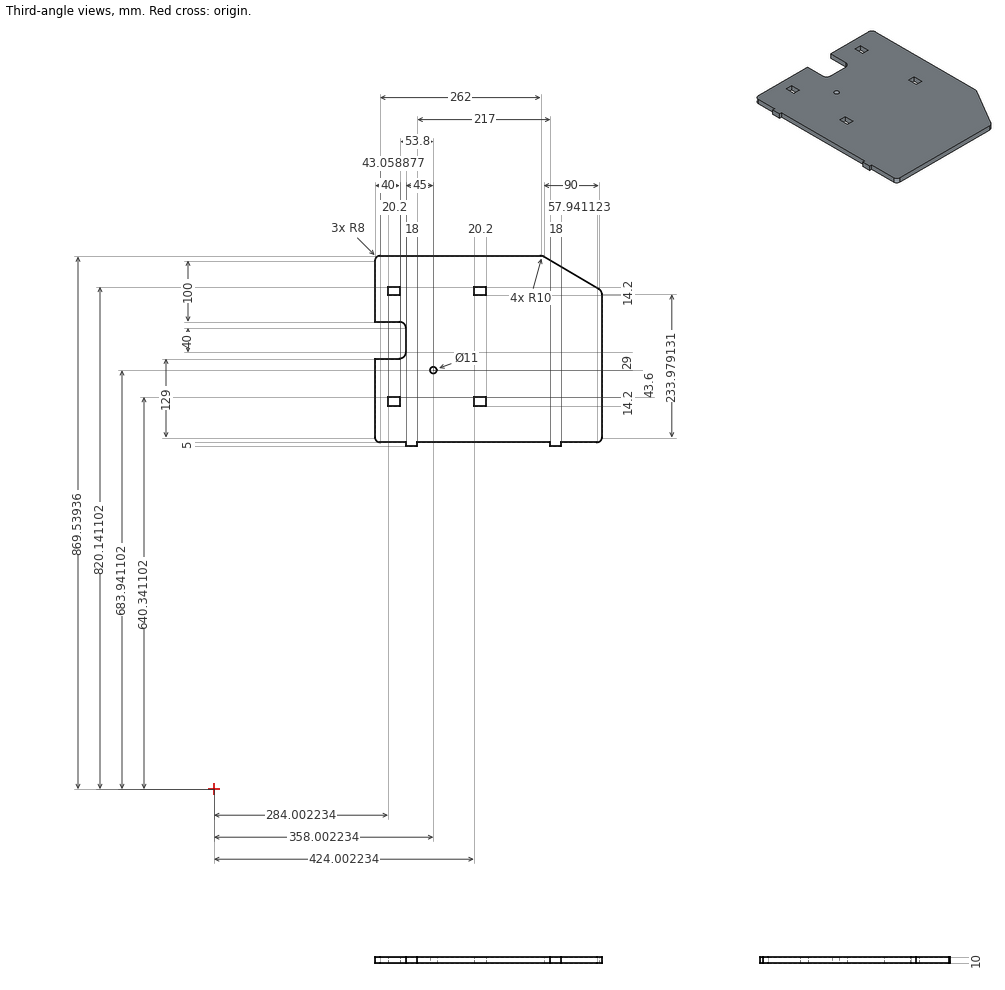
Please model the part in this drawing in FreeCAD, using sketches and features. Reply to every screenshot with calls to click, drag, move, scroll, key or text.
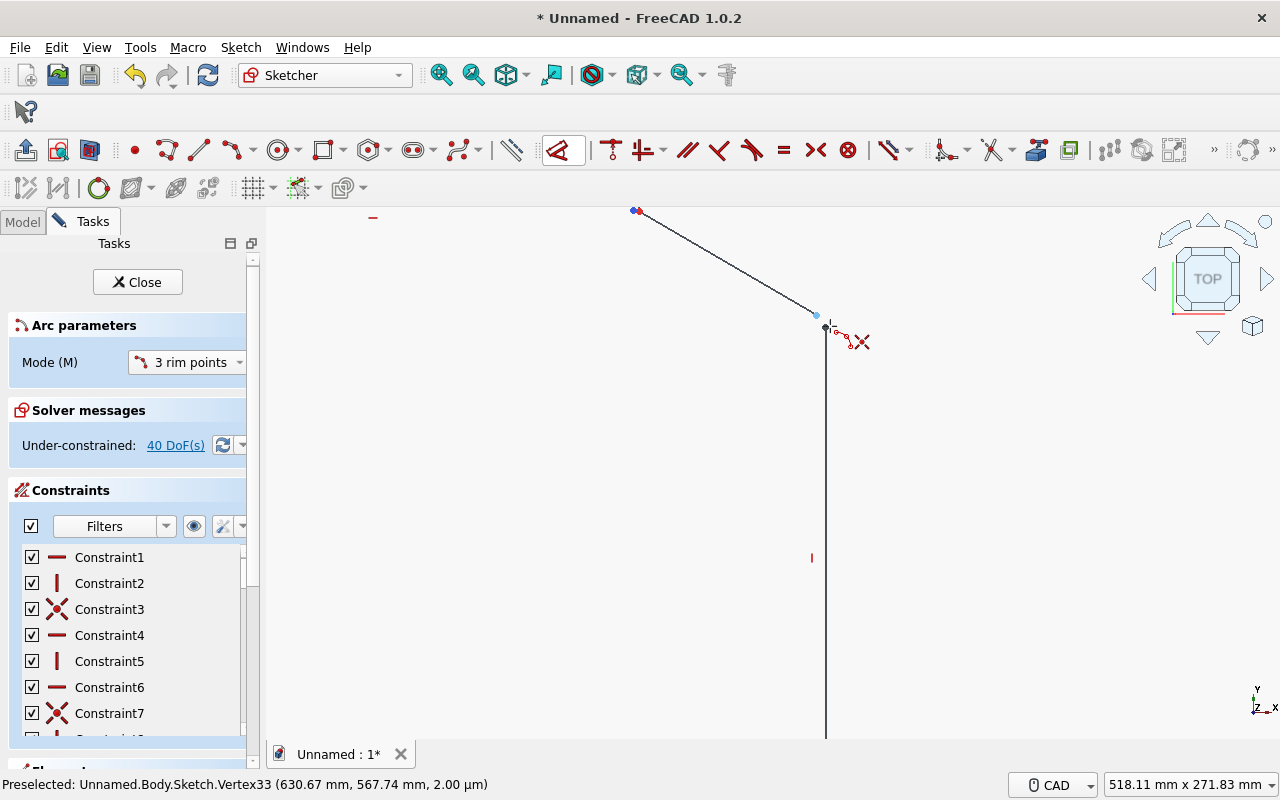
click(826, 328)
click(817, 315)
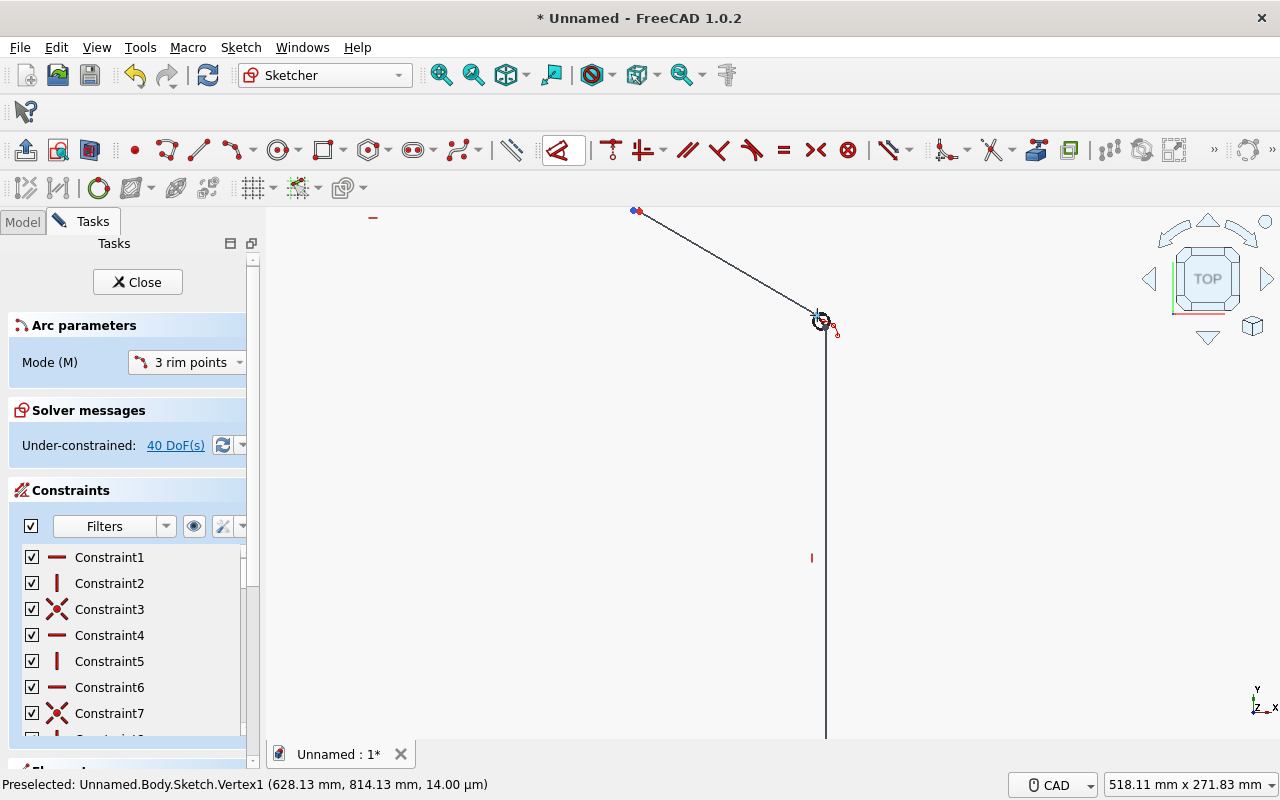
scroll(824, 318, up, 10)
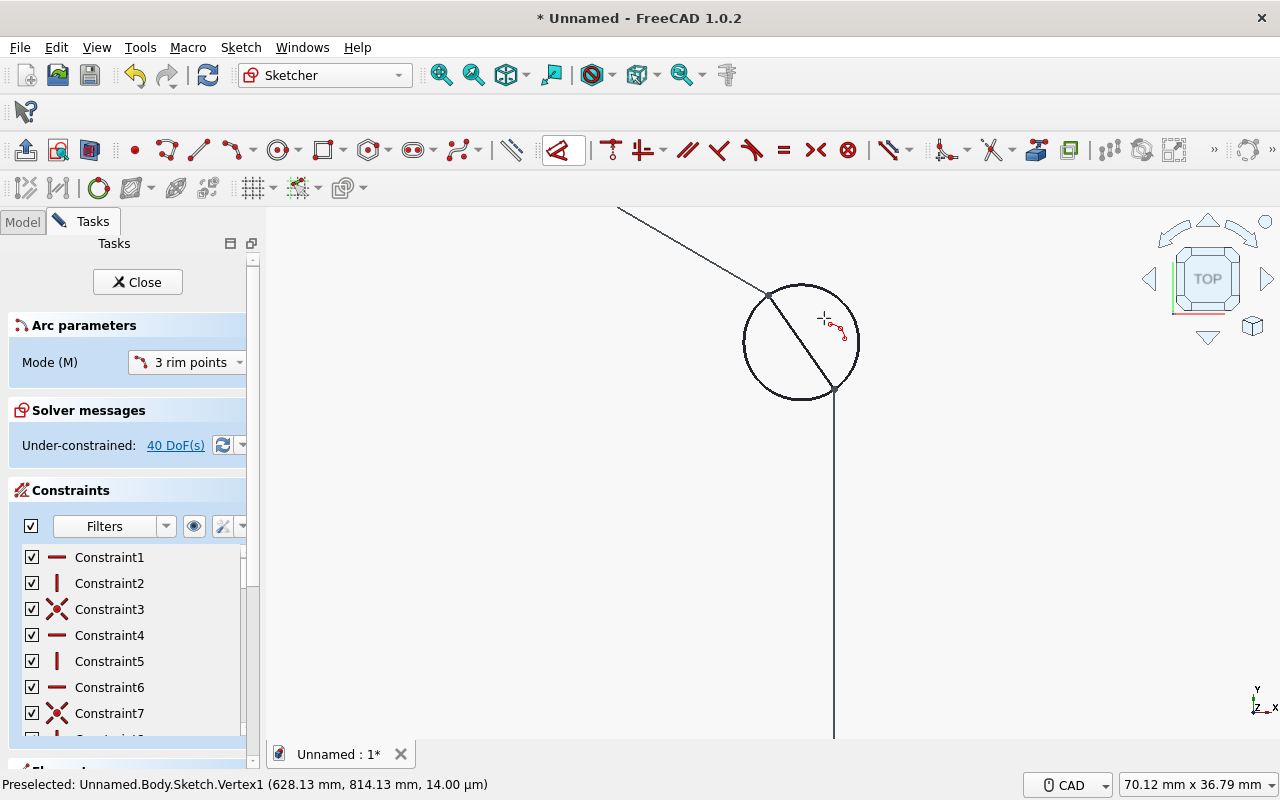
click(820, 313)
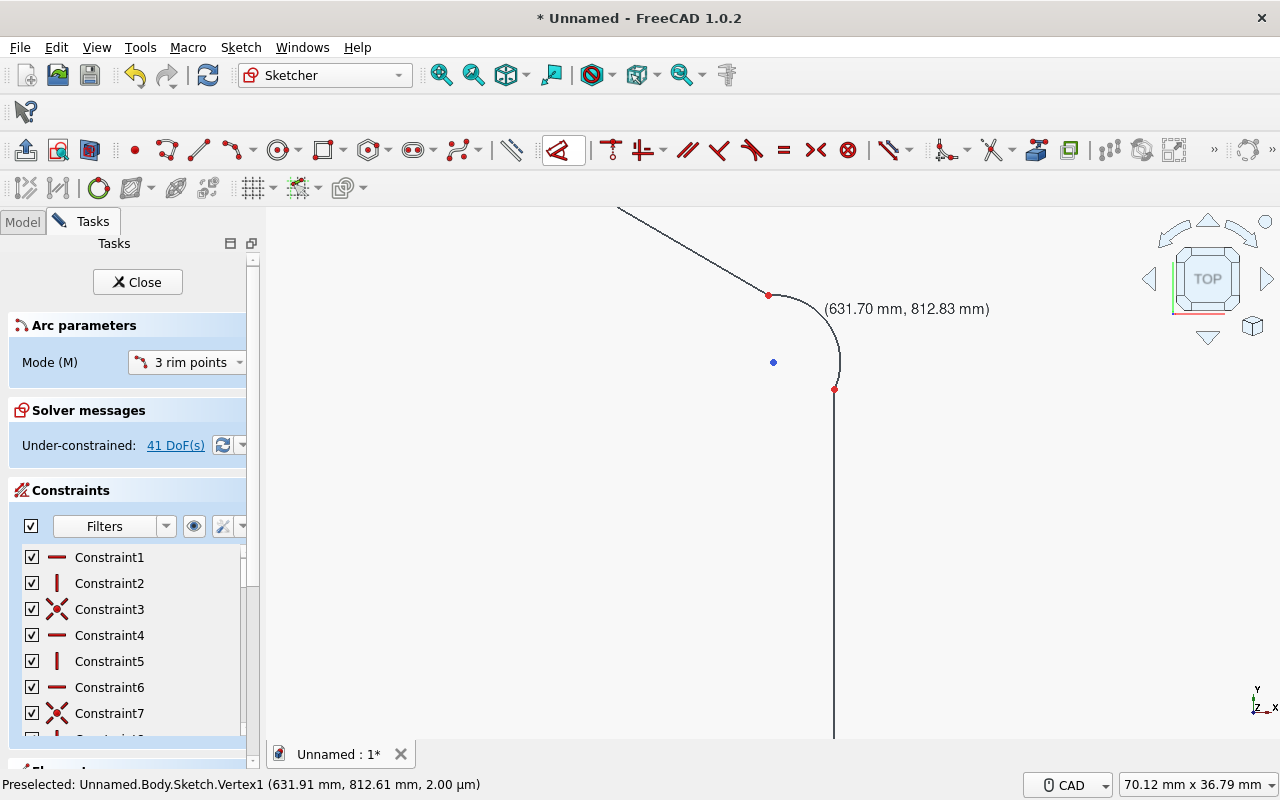
click(324, 150)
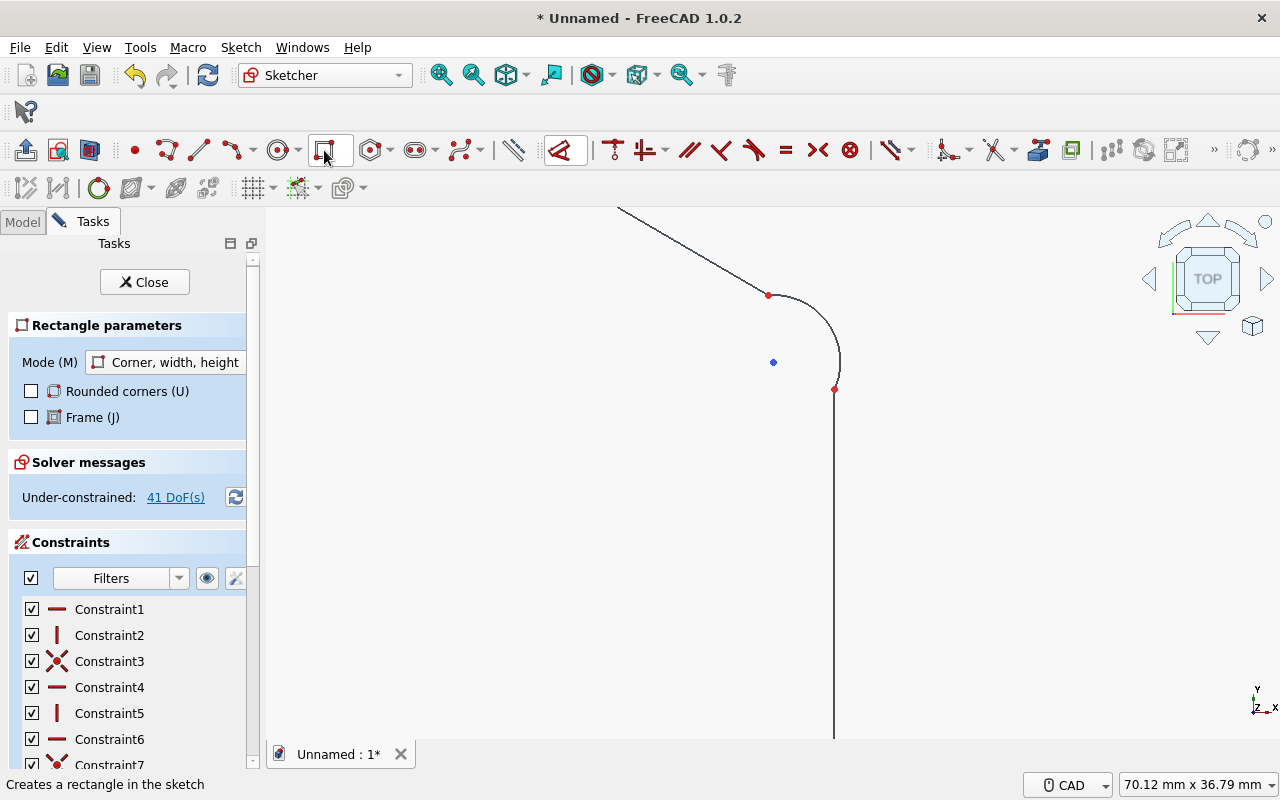
scroll(858, 290, down, 17)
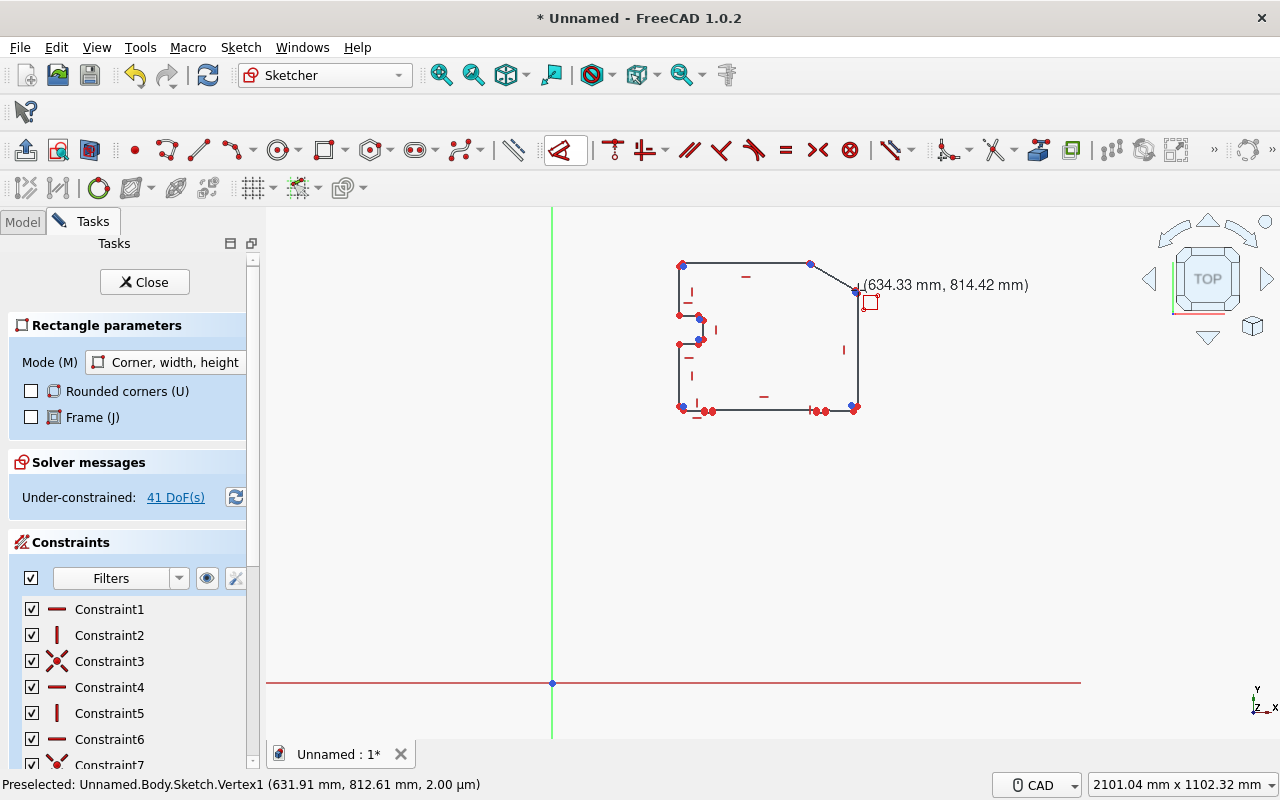
scroll(757, 374, up, 5)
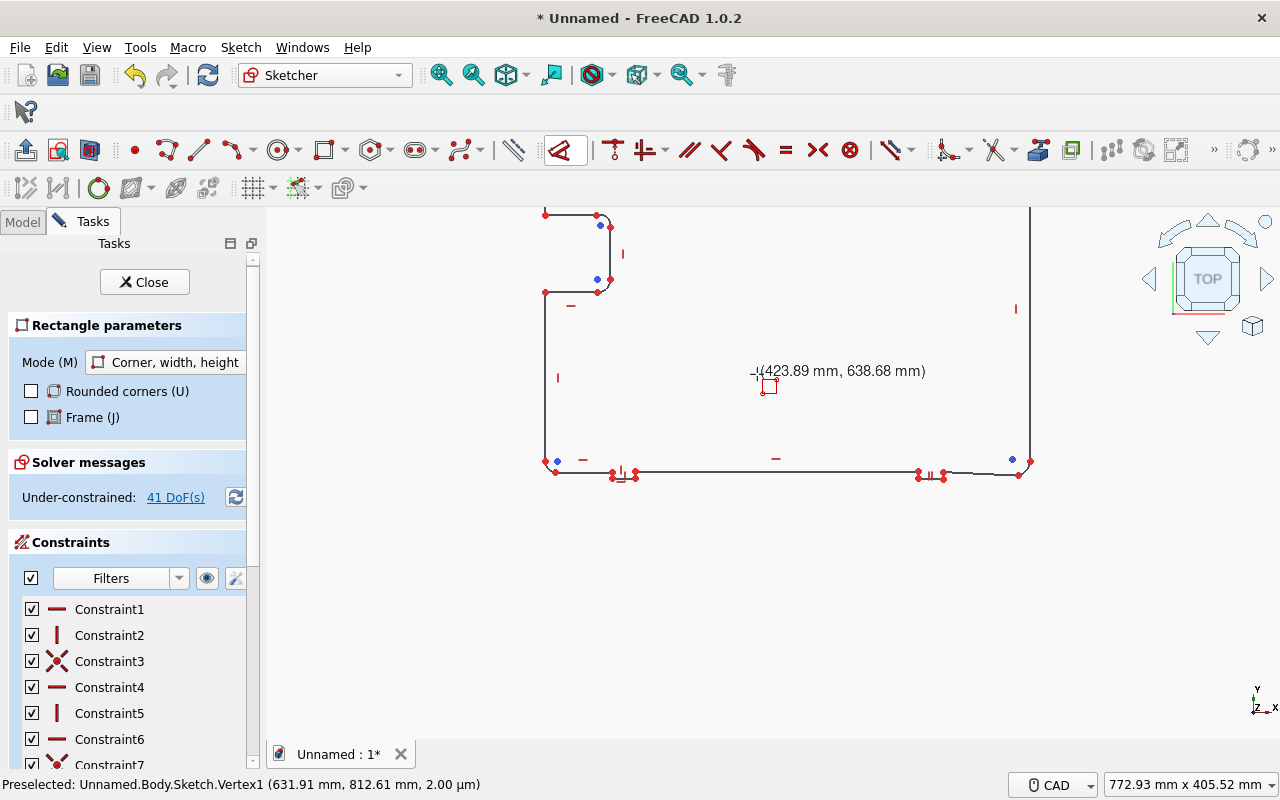
click(756, 374)
move(783, 393)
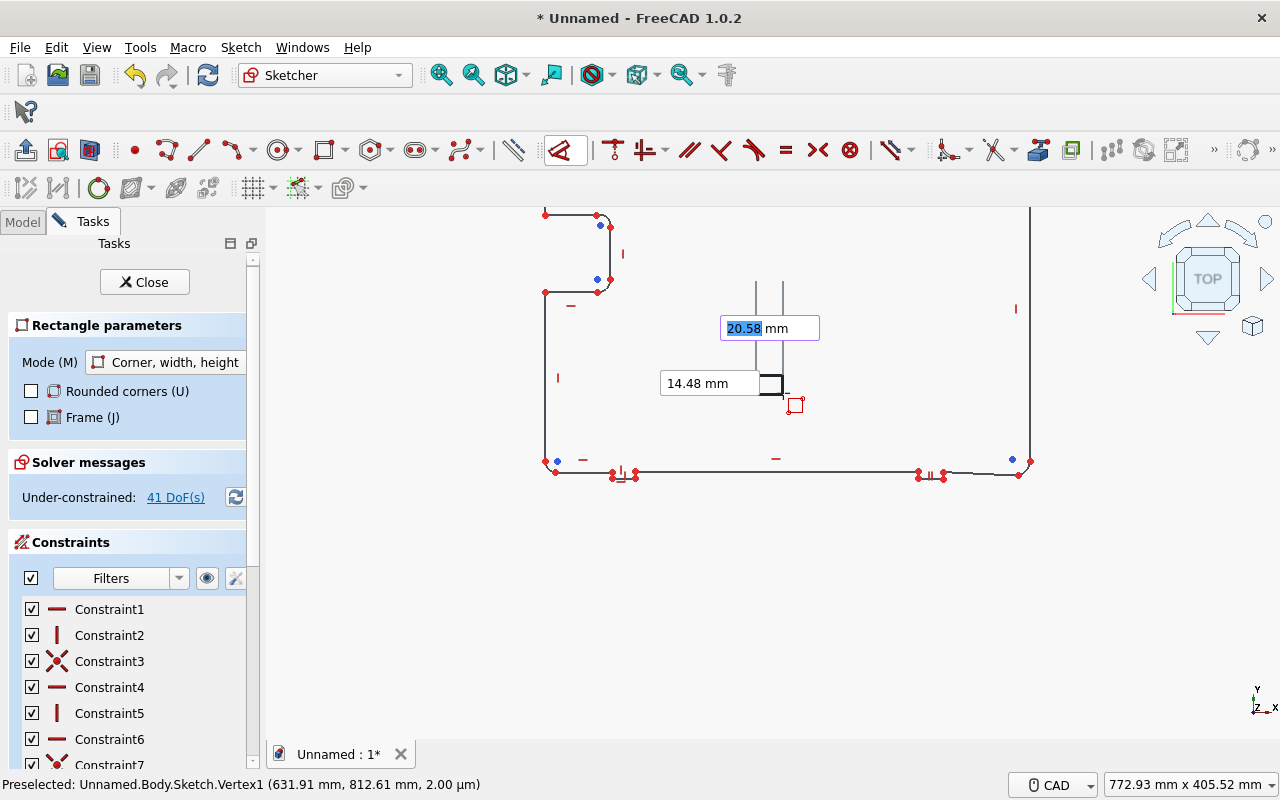
text(20.2)
key(Tab)
text(14.2)
key(Return)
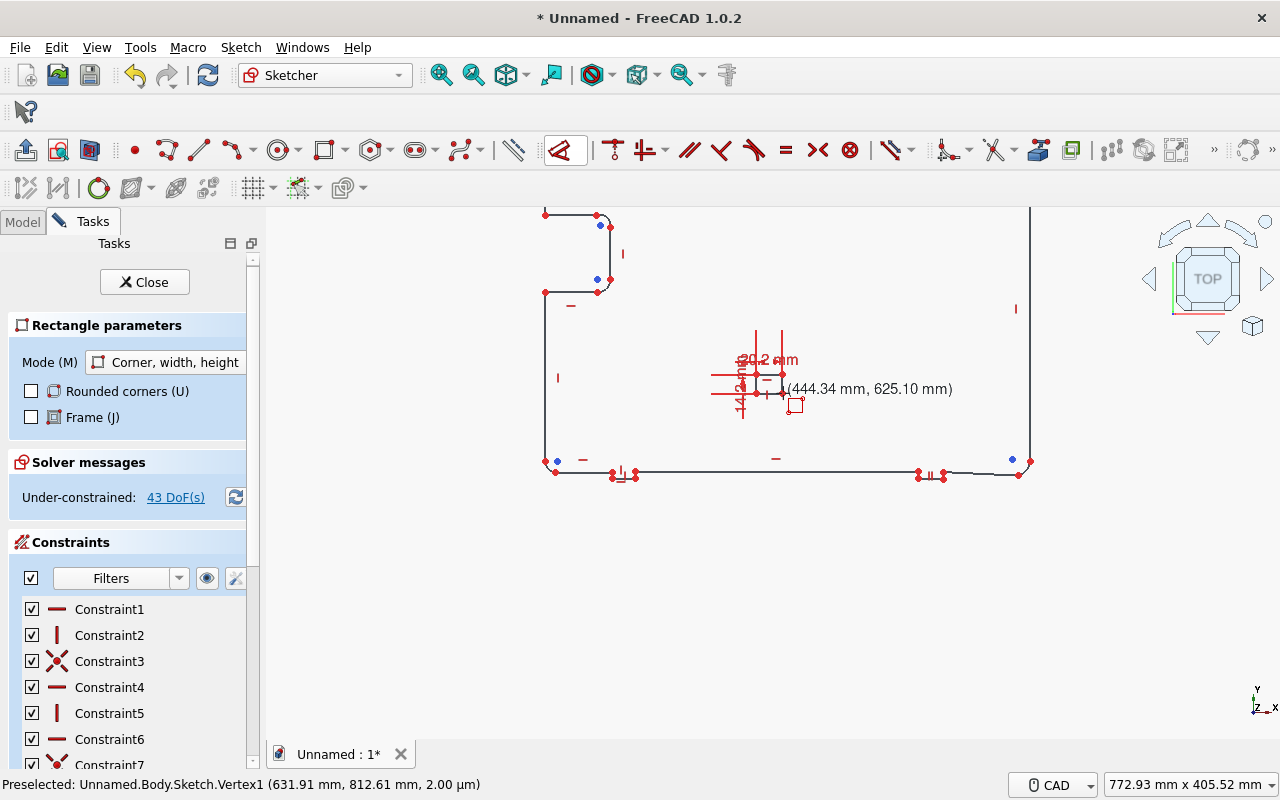
click(573, 374)
move(599, 393)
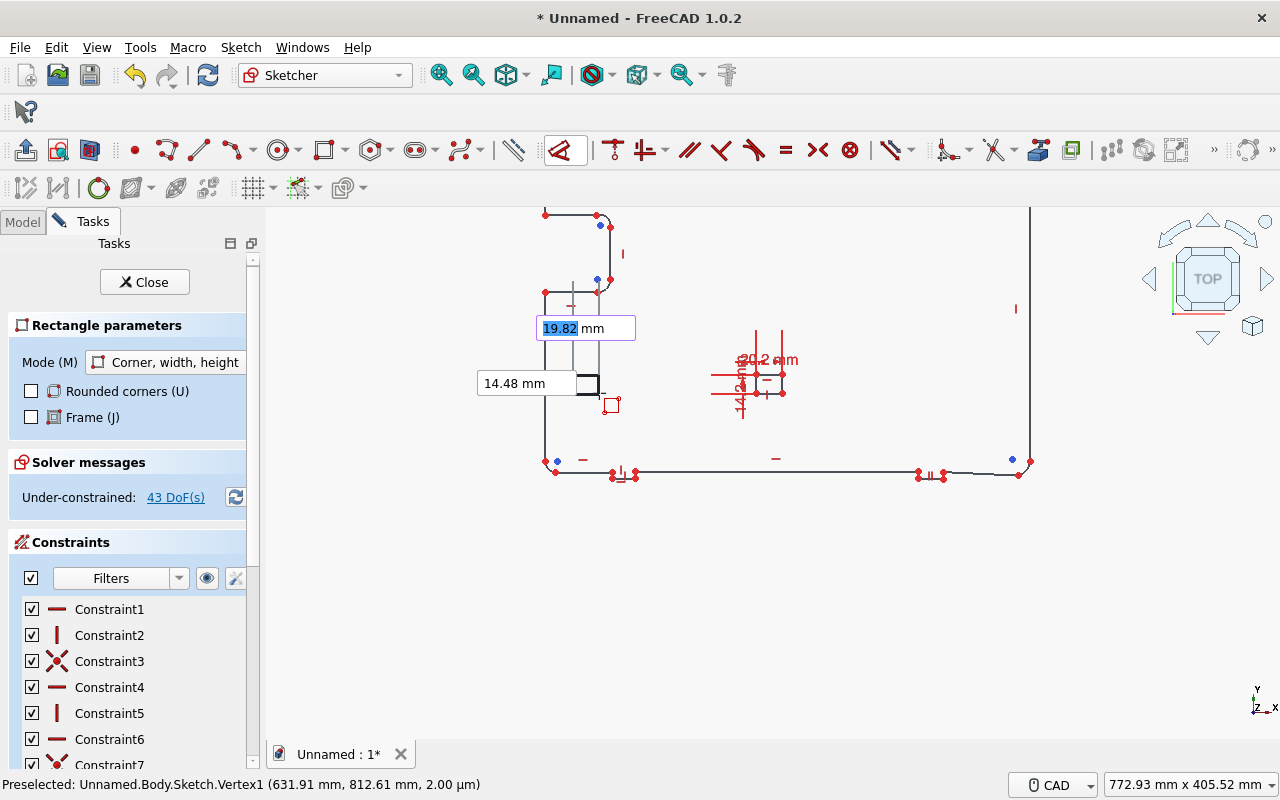
text(20.2)
key(Tab)
text(14.2)
key(Return)